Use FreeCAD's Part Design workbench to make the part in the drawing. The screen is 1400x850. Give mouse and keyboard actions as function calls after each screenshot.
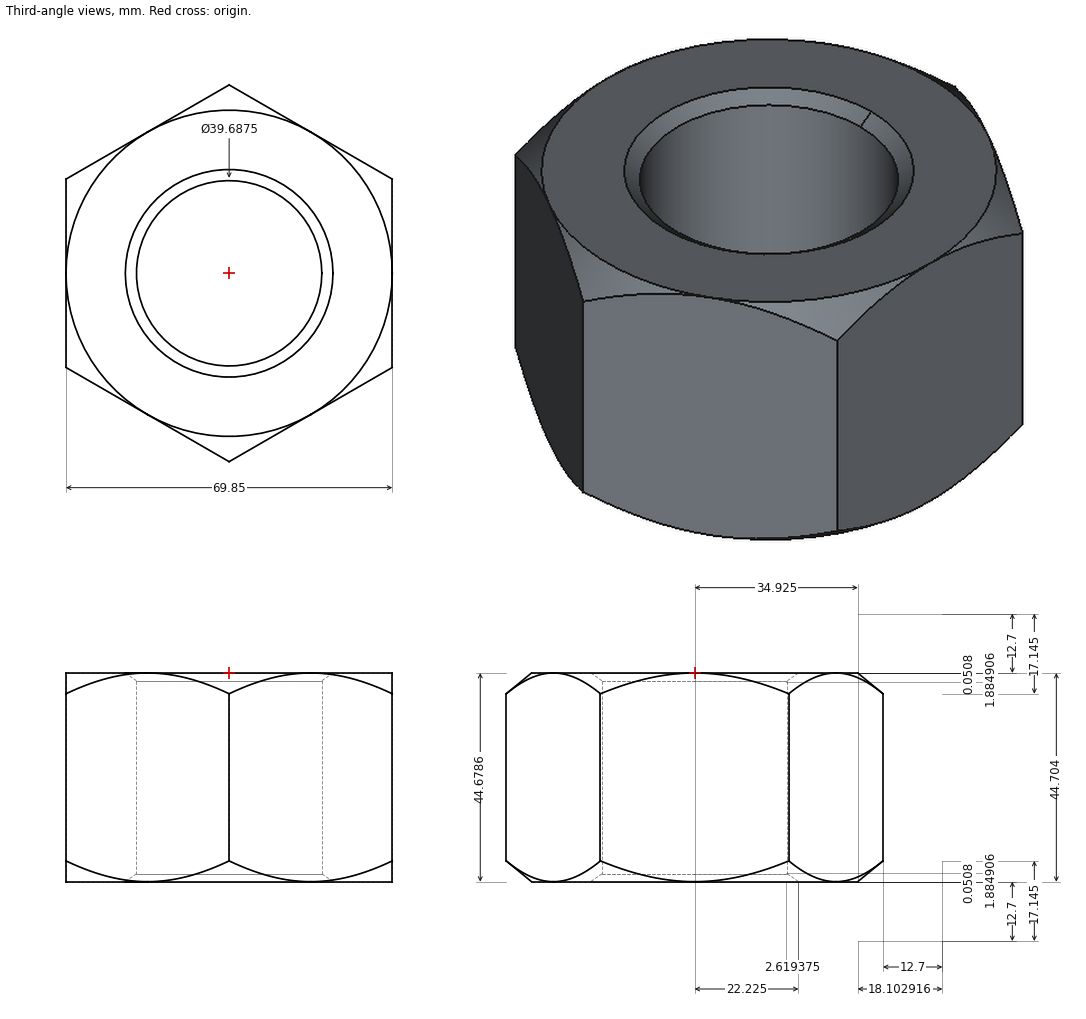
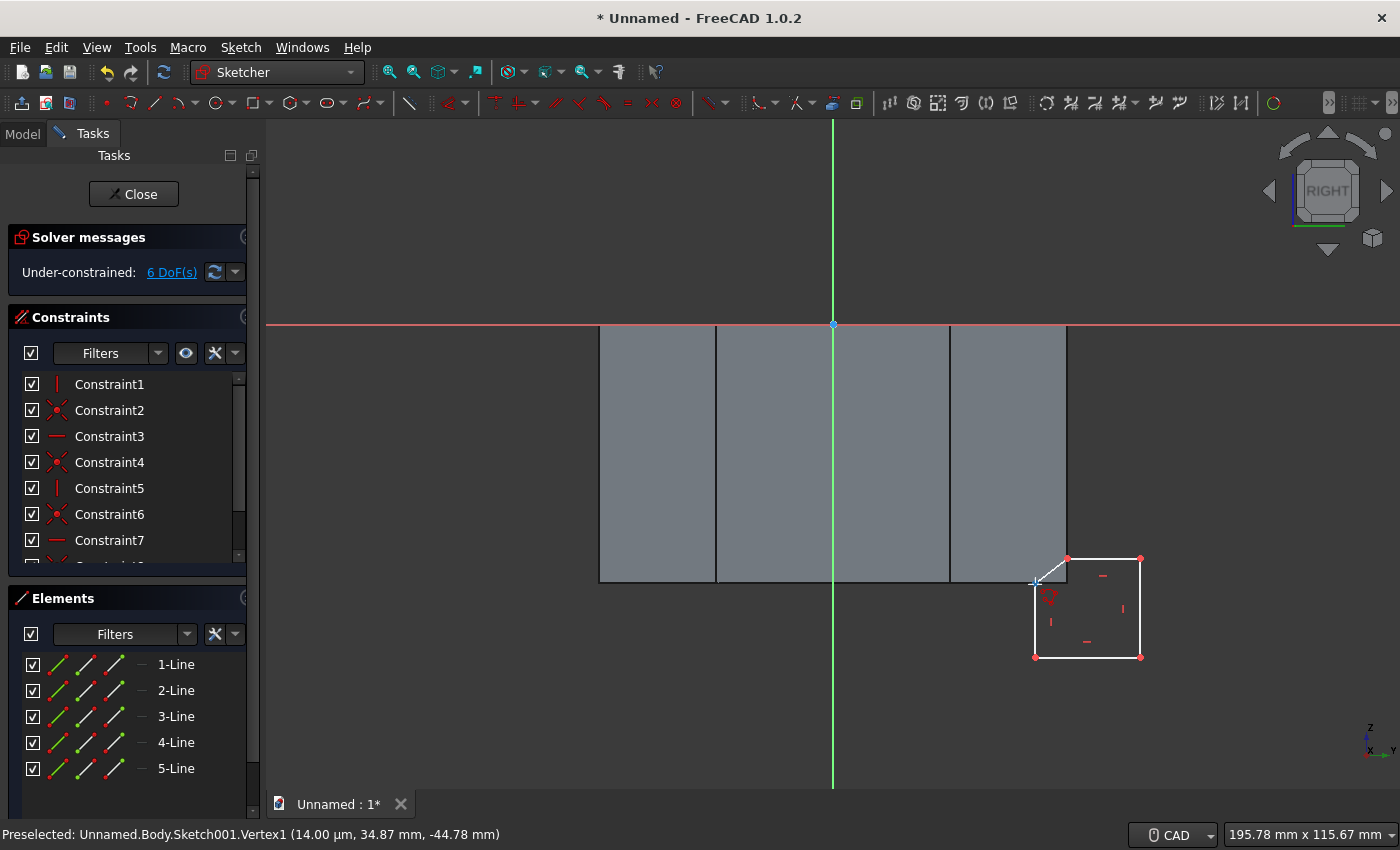
click(1035, 325)
click(1067, 350)
click(1140, 350)
click(1140, 251)
click(1035, 251)
click(1035, 325)
key(Escape)
key(Escape)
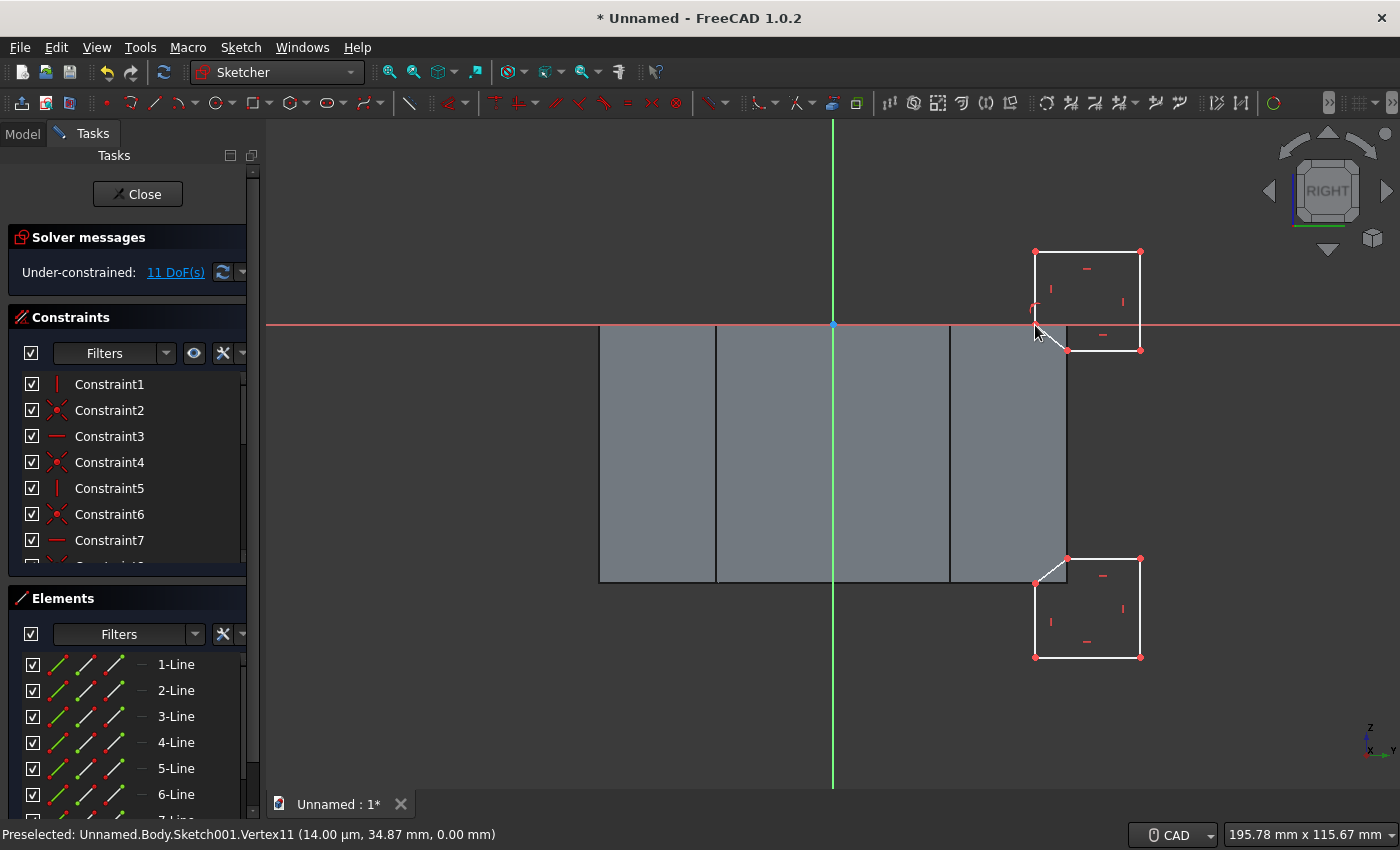
click(448, 104)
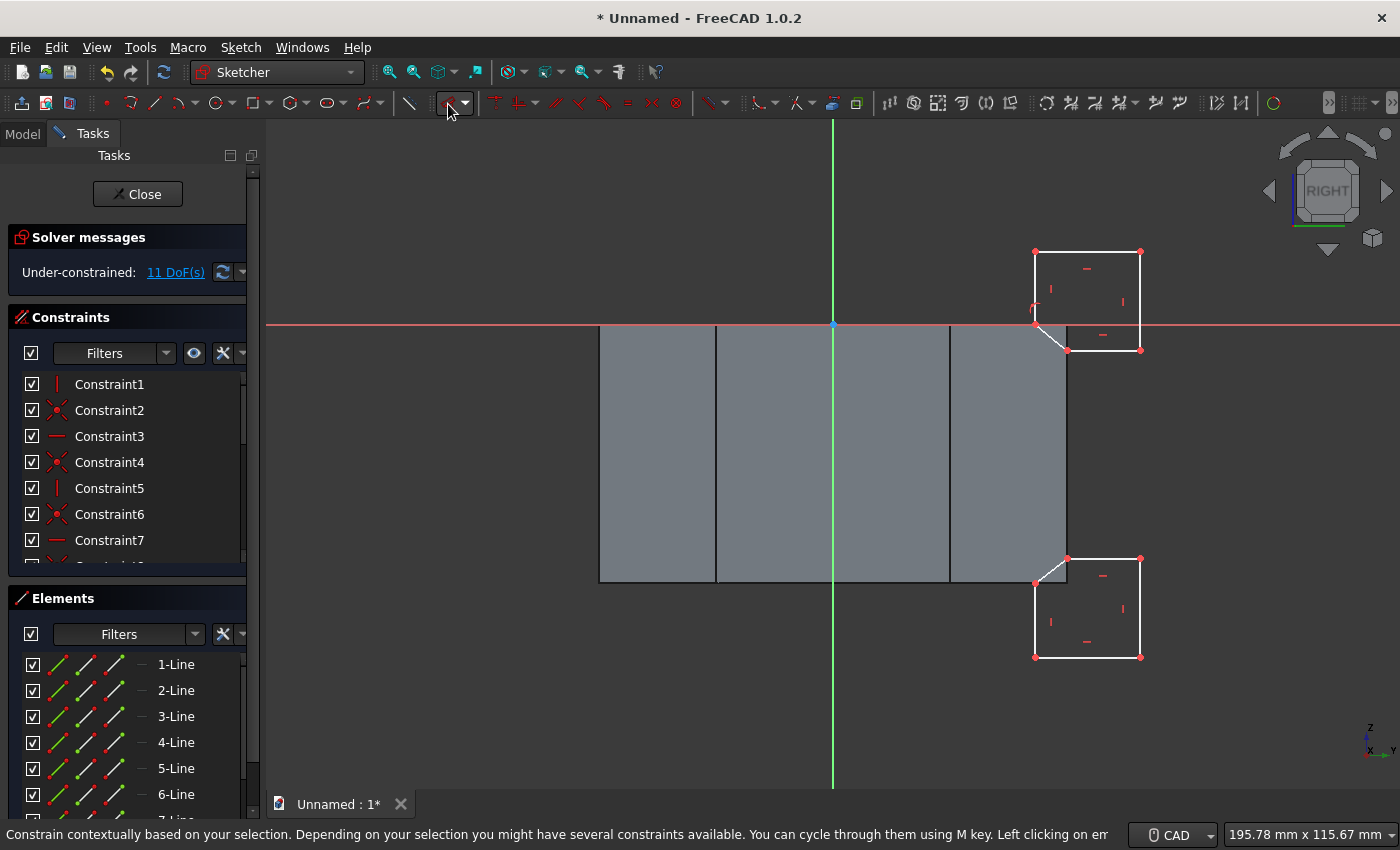
click(1035, 606)
click(1069, 621)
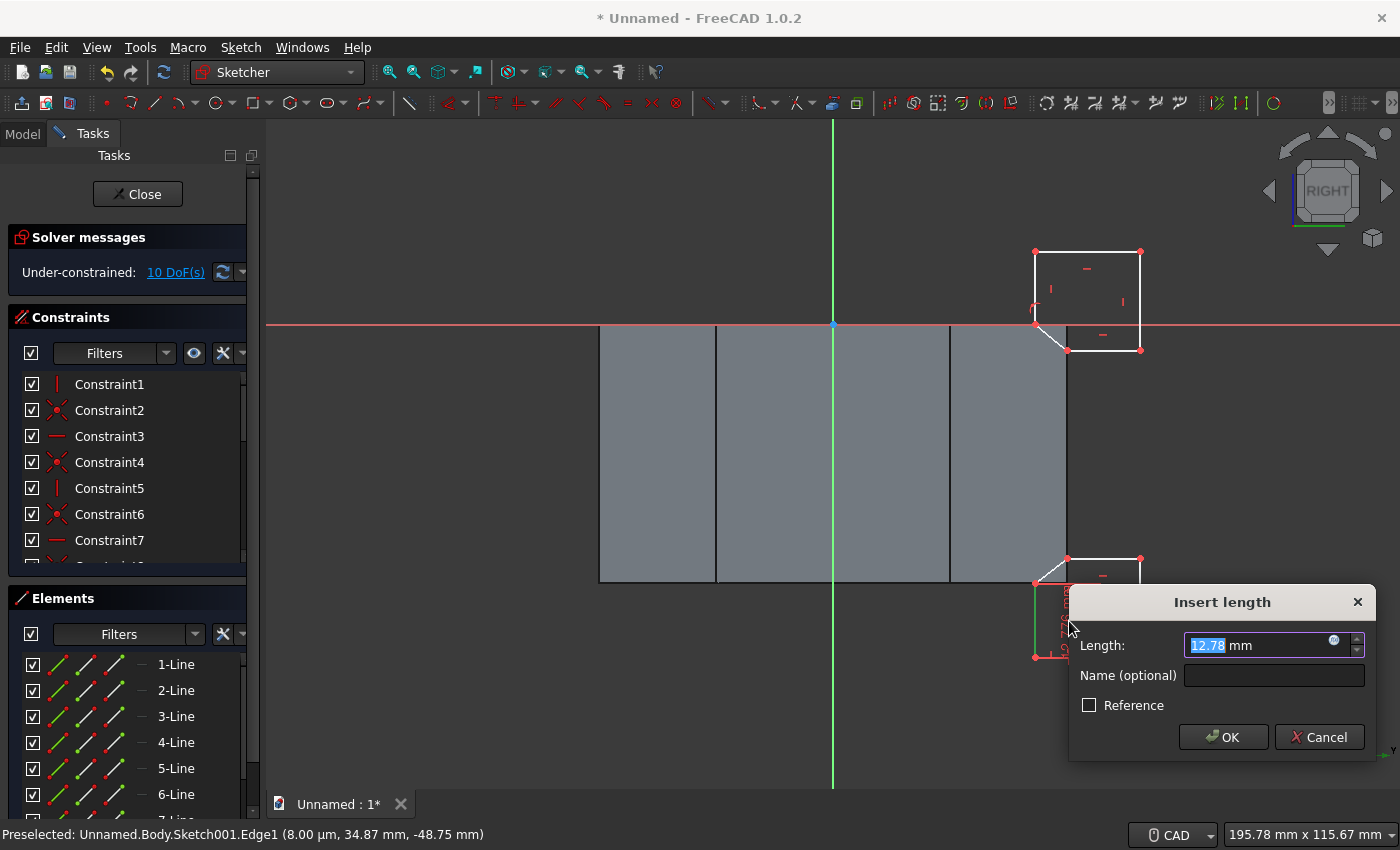
text(12.7)
key(Return)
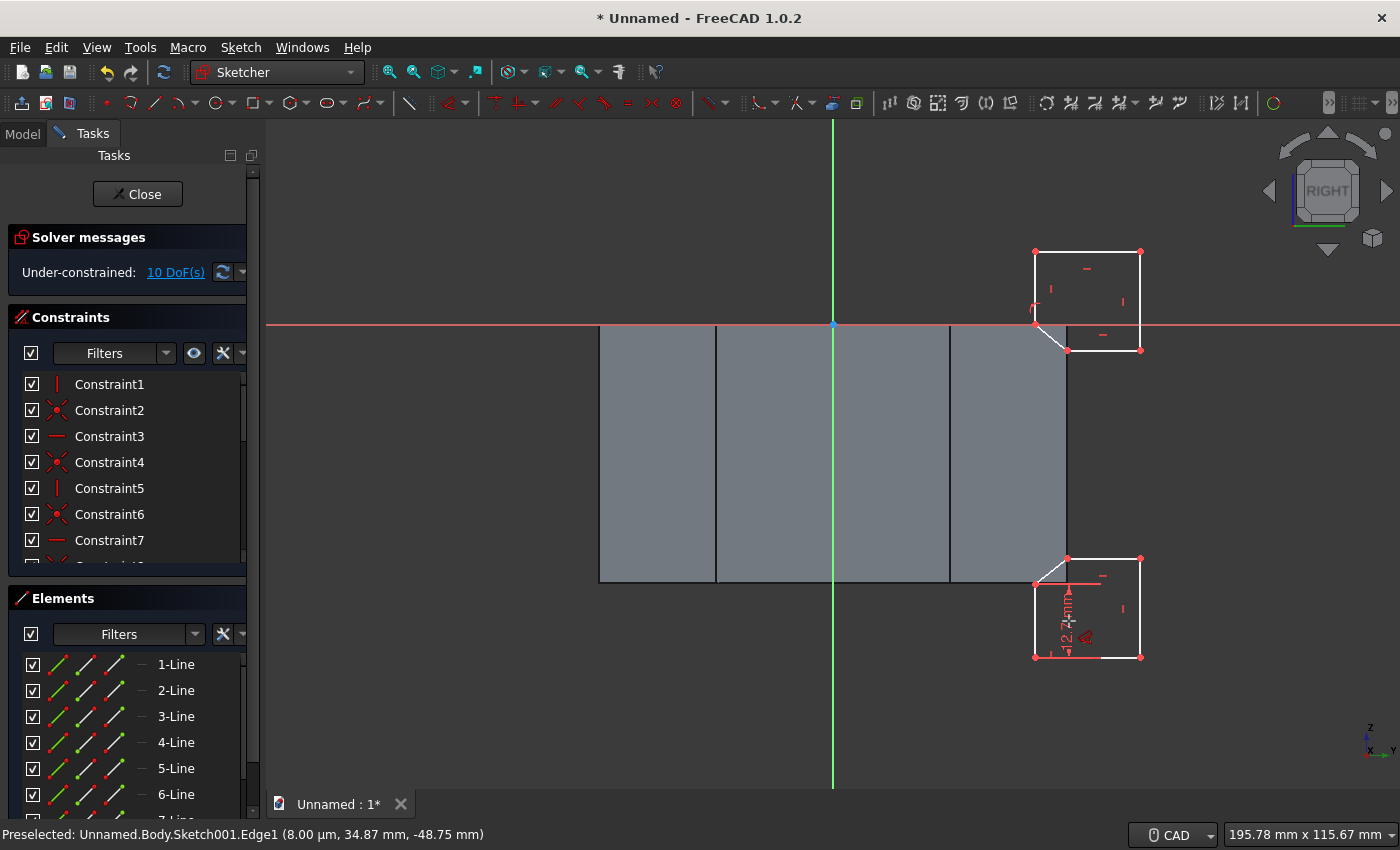
click(1118, 559)
click(1103, 593)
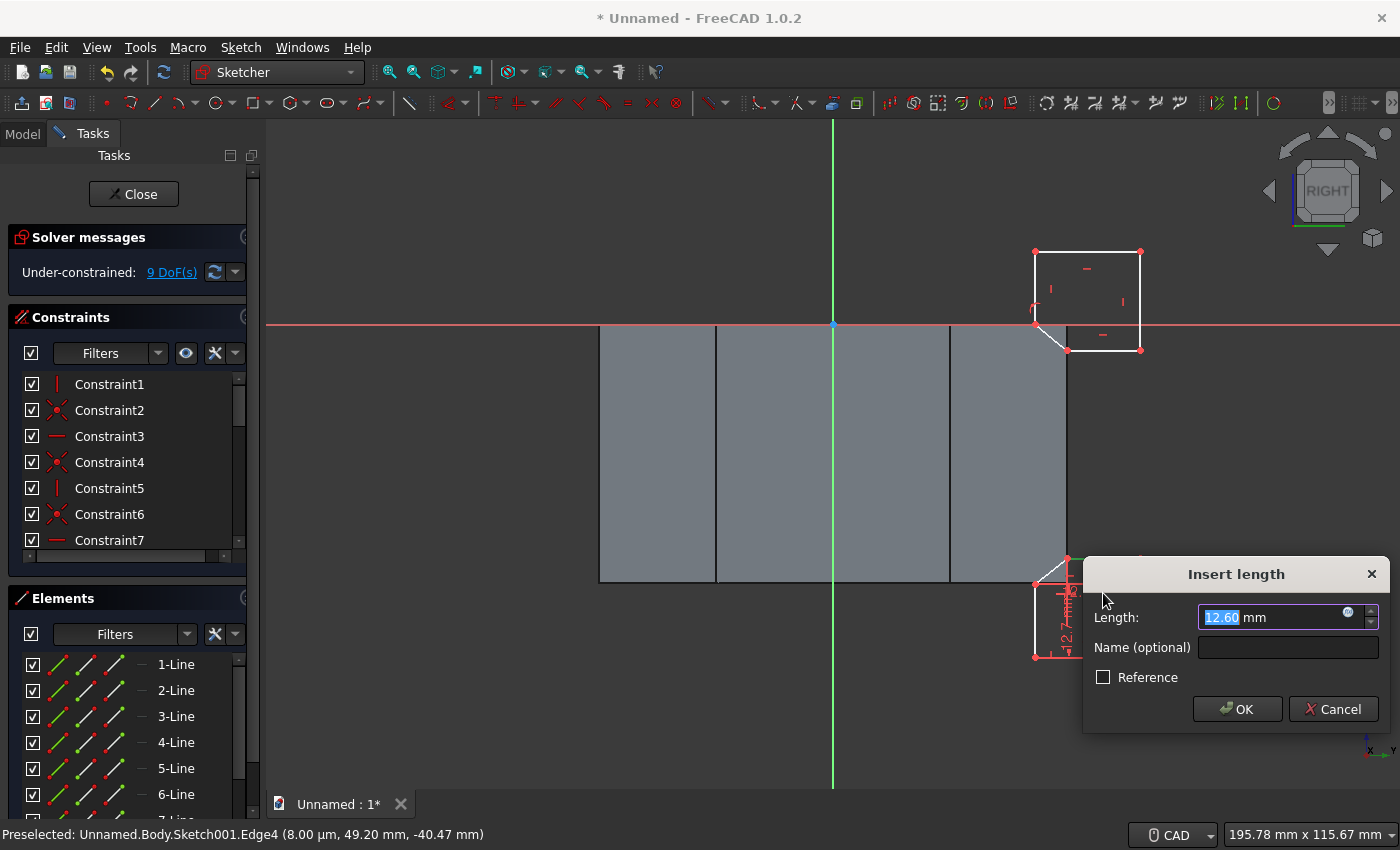
text(12.7)
key(Return)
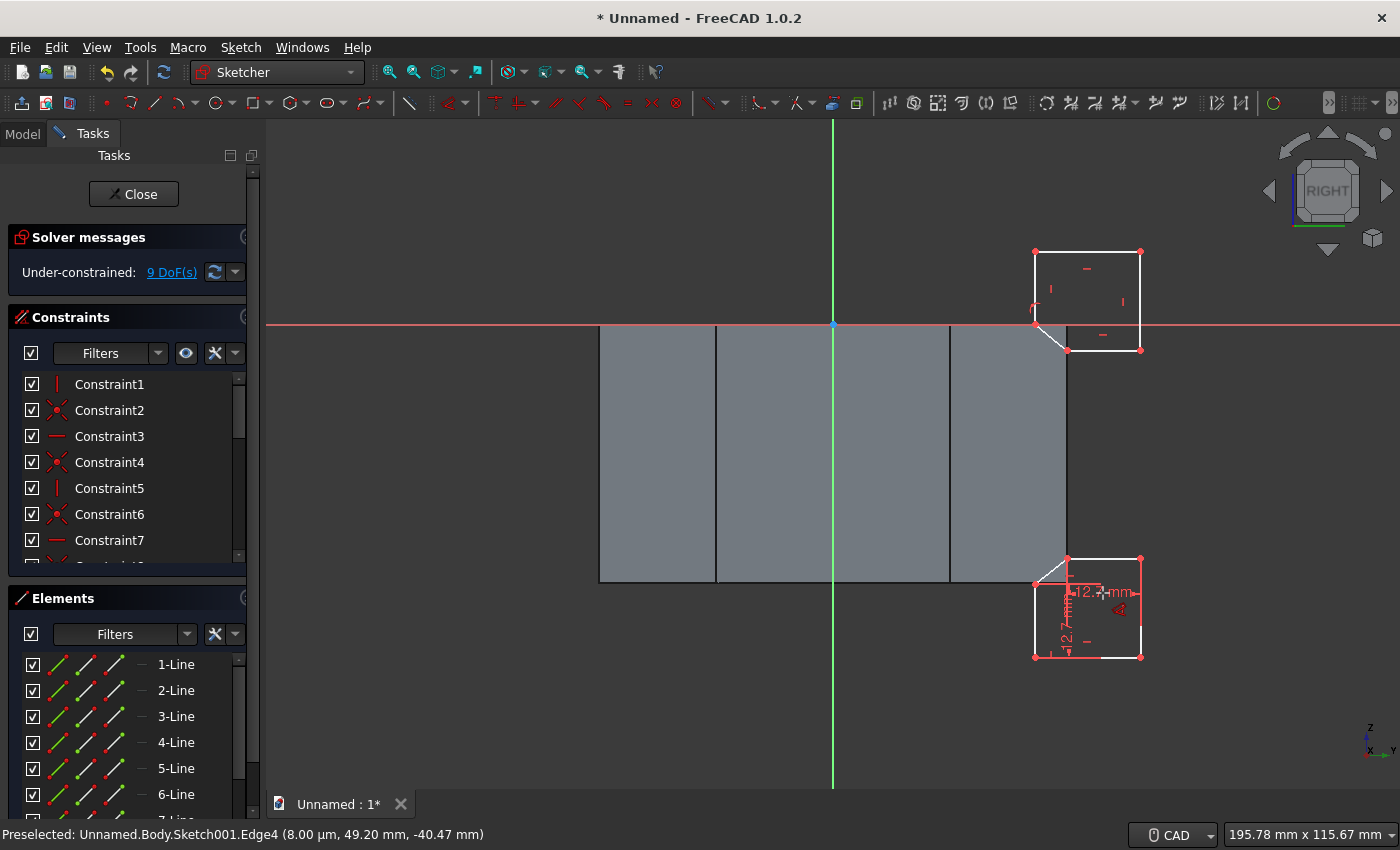
click(1089, 351)
click(1103, 385)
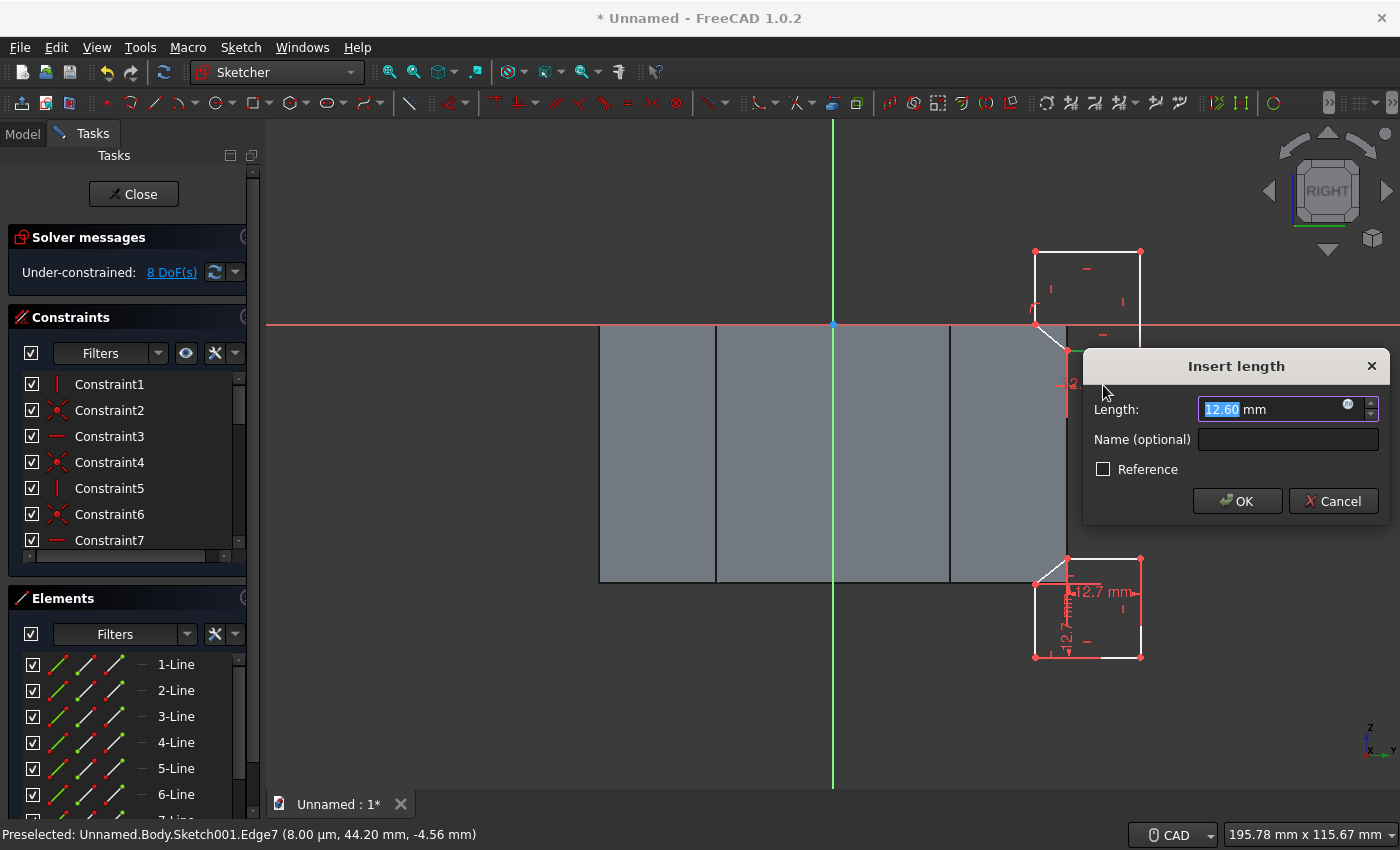
text(12.7)
key(Return)